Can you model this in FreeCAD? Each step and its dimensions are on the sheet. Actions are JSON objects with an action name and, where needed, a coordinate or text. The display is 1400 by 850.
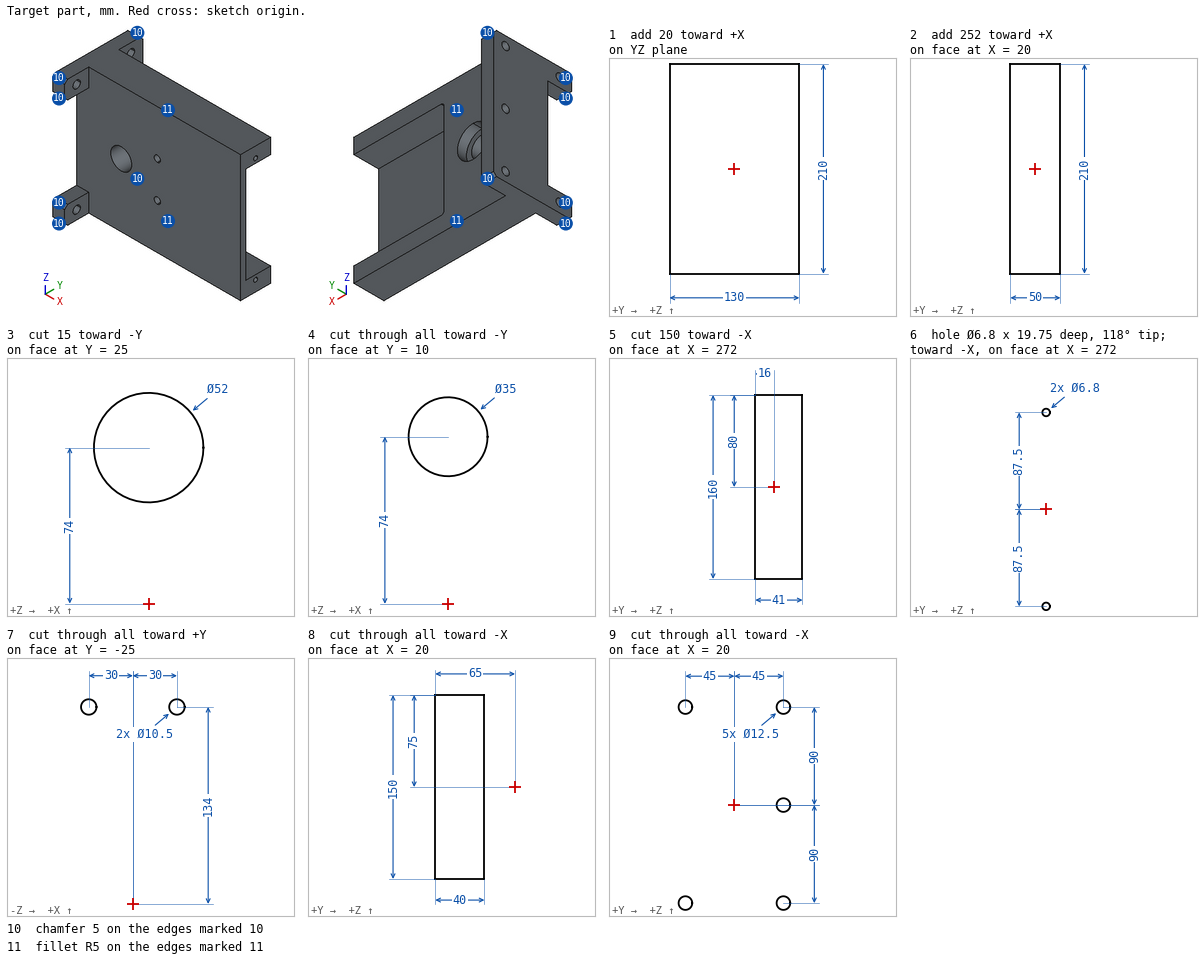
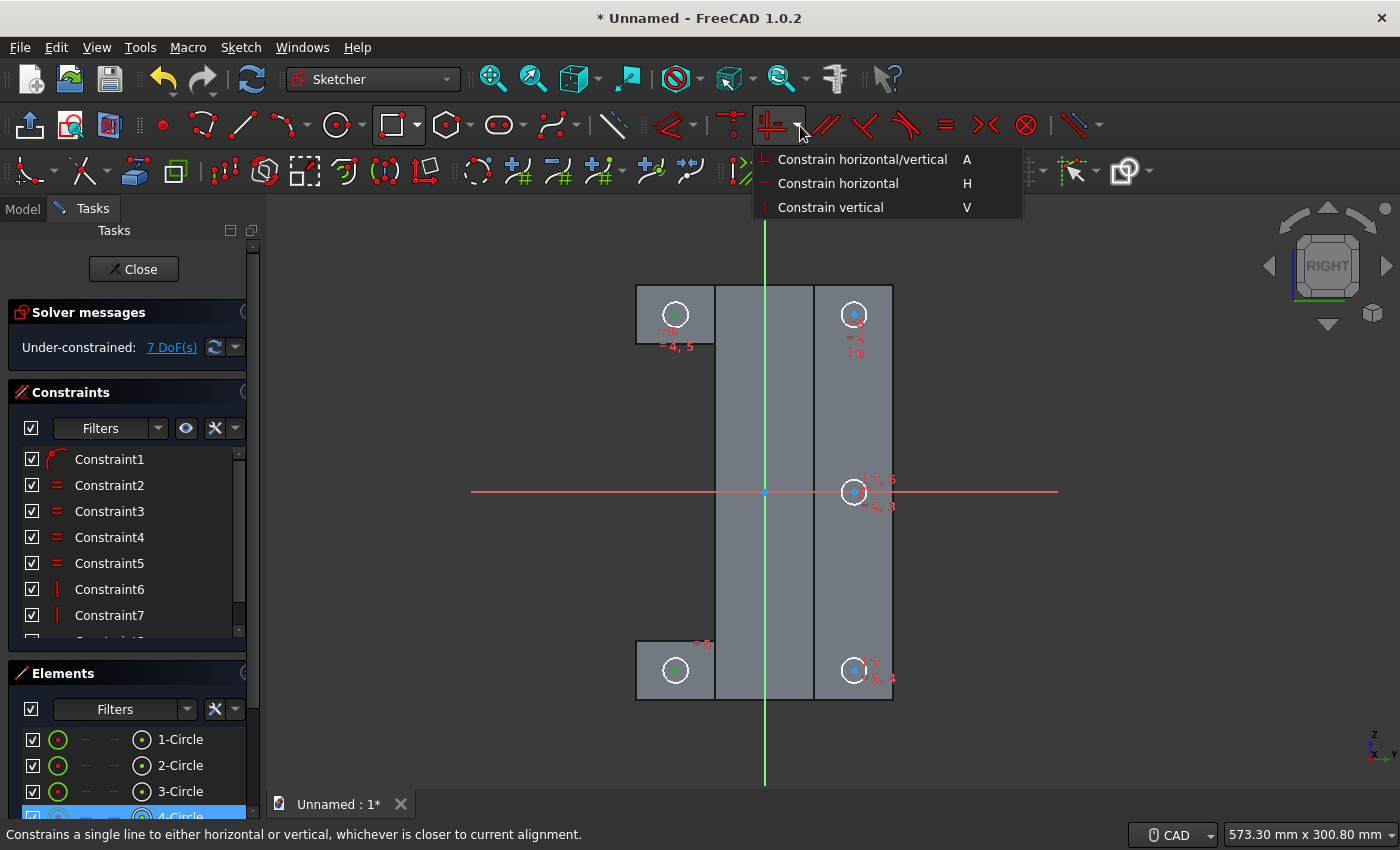
{"action": "left_click", "coordinate": [888, 207]}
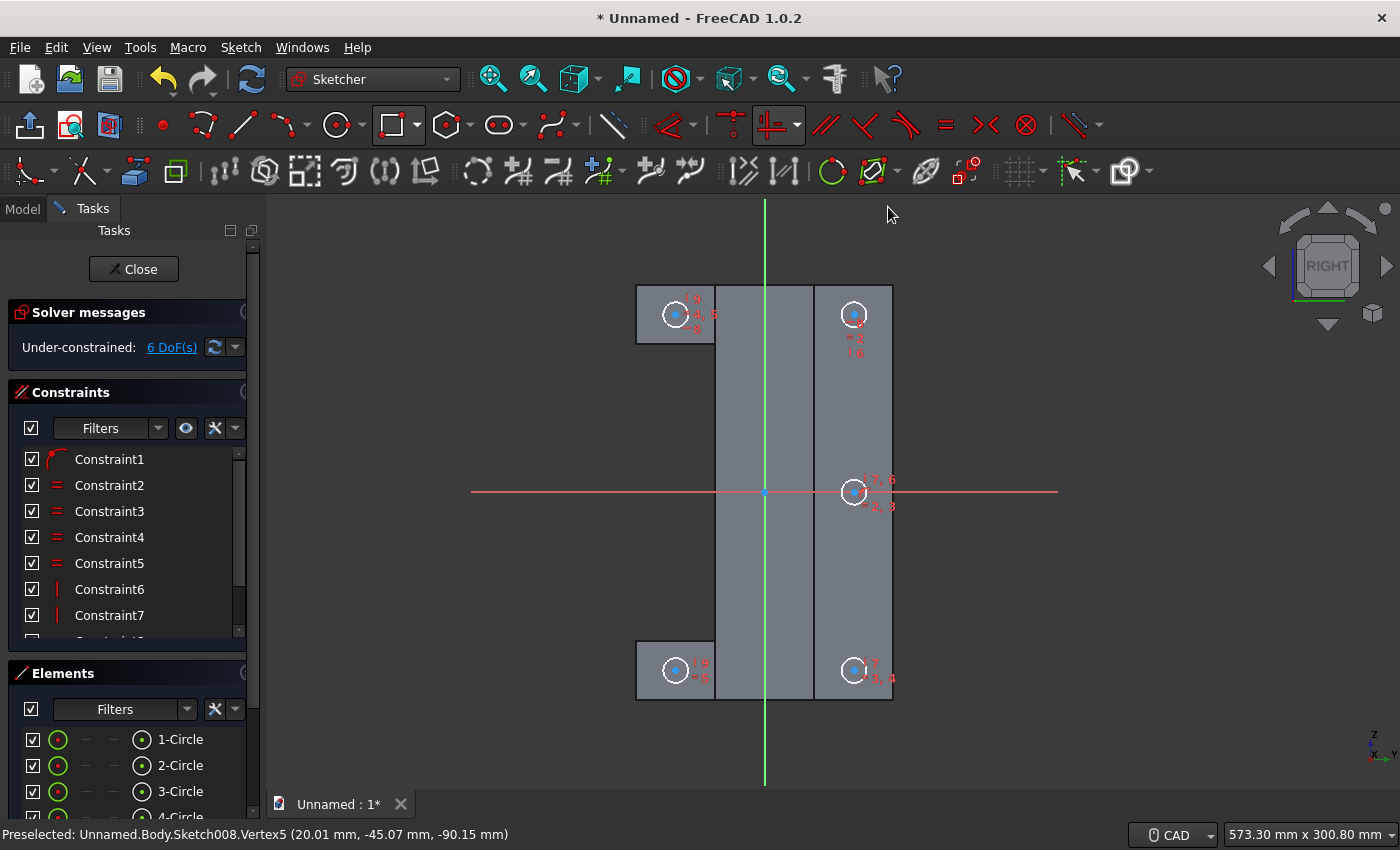
{"action": "left_click", "coordinate": [854, 671]}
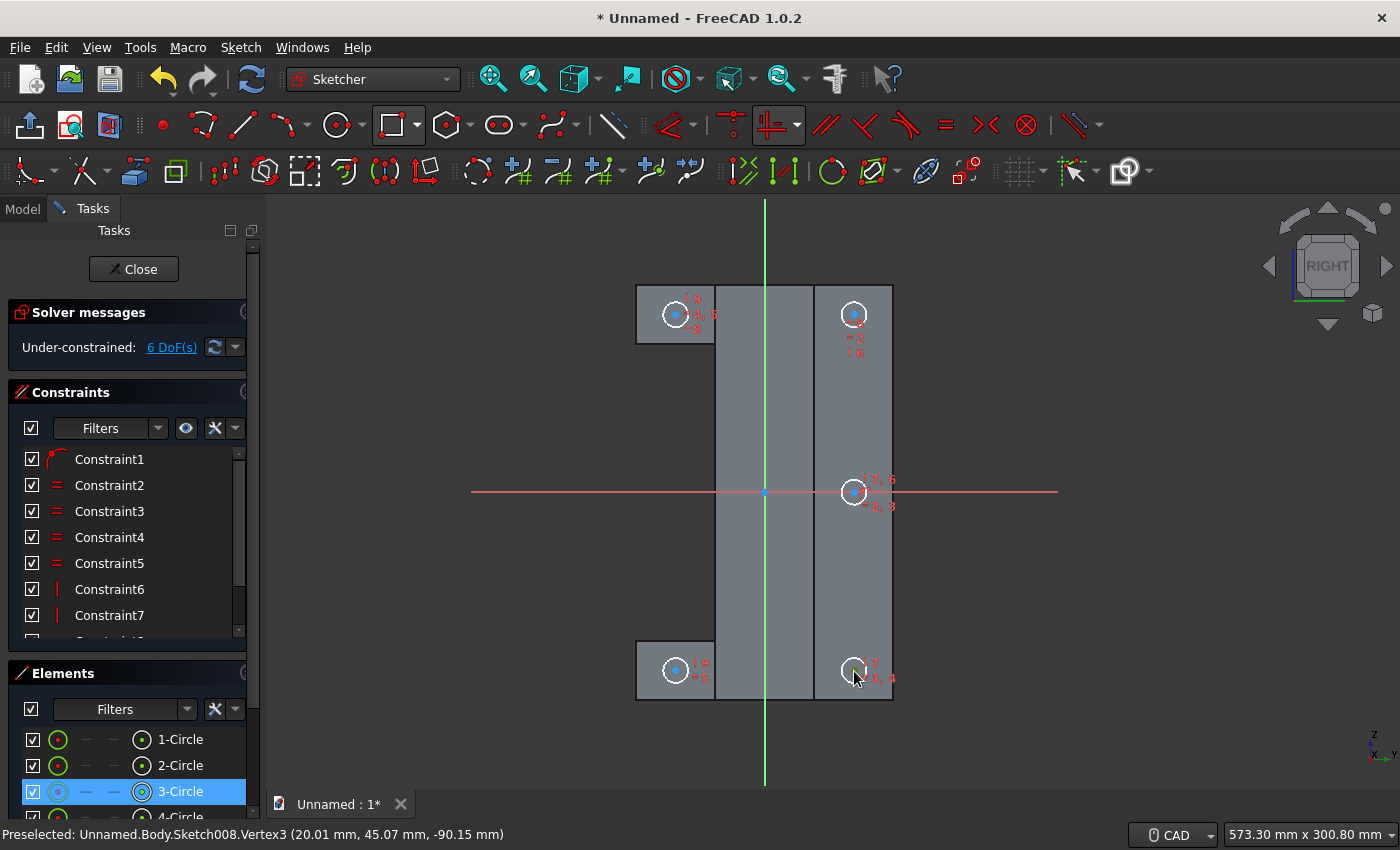
{"action": "left_click", "coordinate": [676, 671]}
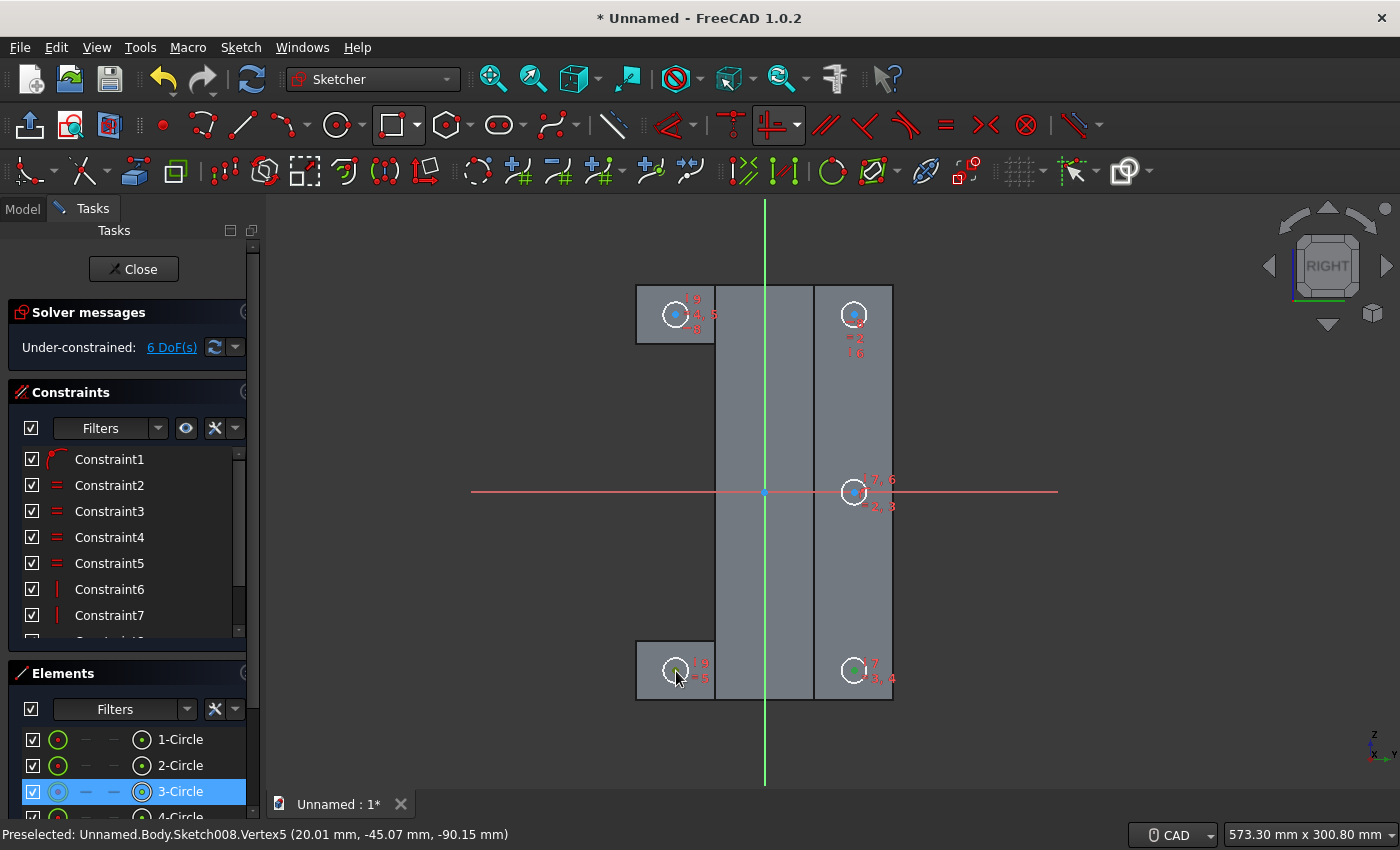
{"action": "left_click", "coordinate": [800, 126]}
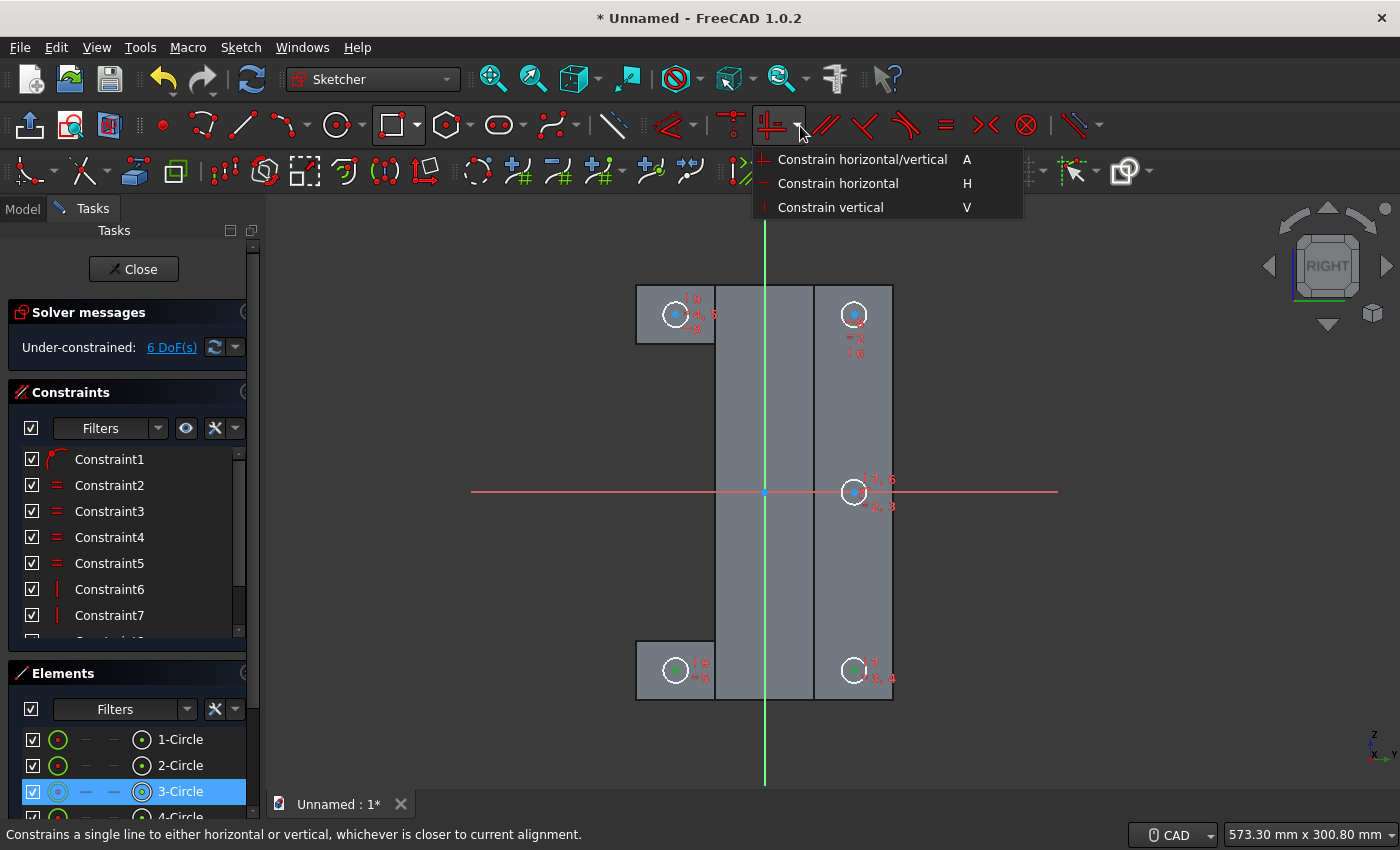
{"action": "left_click", "coordinate": [888, 183]}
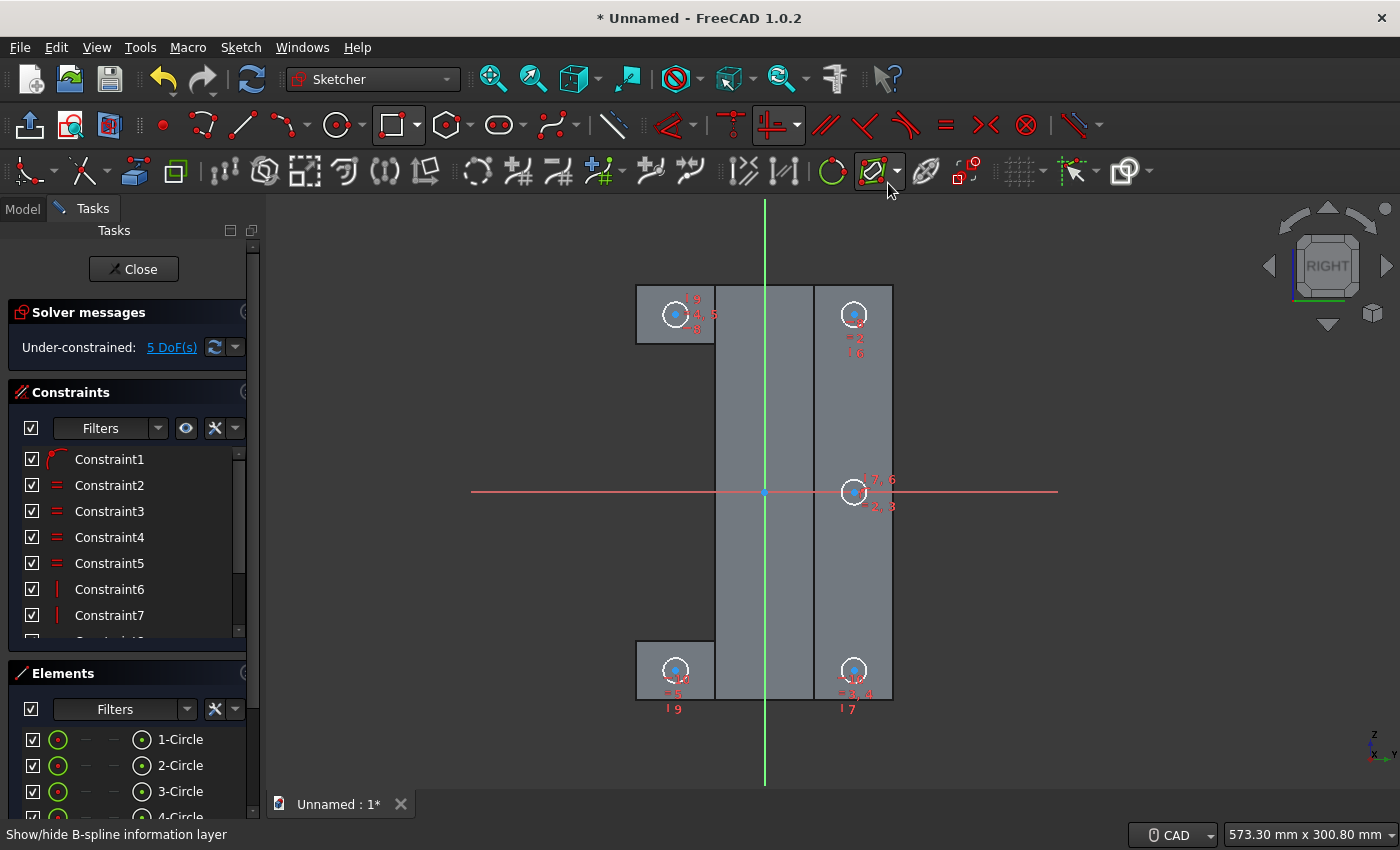
{"action": "left_click", "coordinate": [668, 126]}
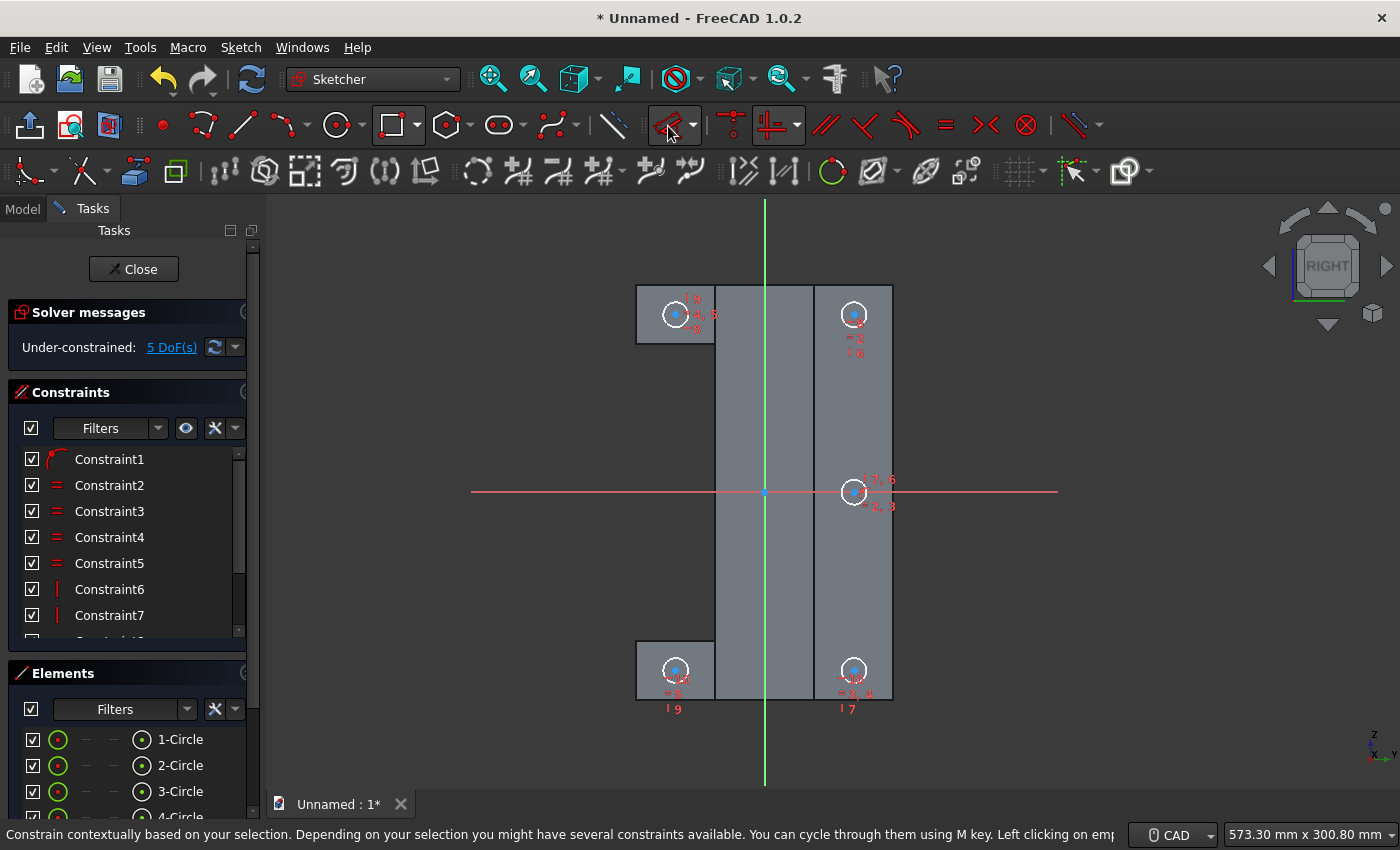
{"action": "scroll", "coordinate": [863, 306], "scroll_direction": "up", "scroll_amount": 3}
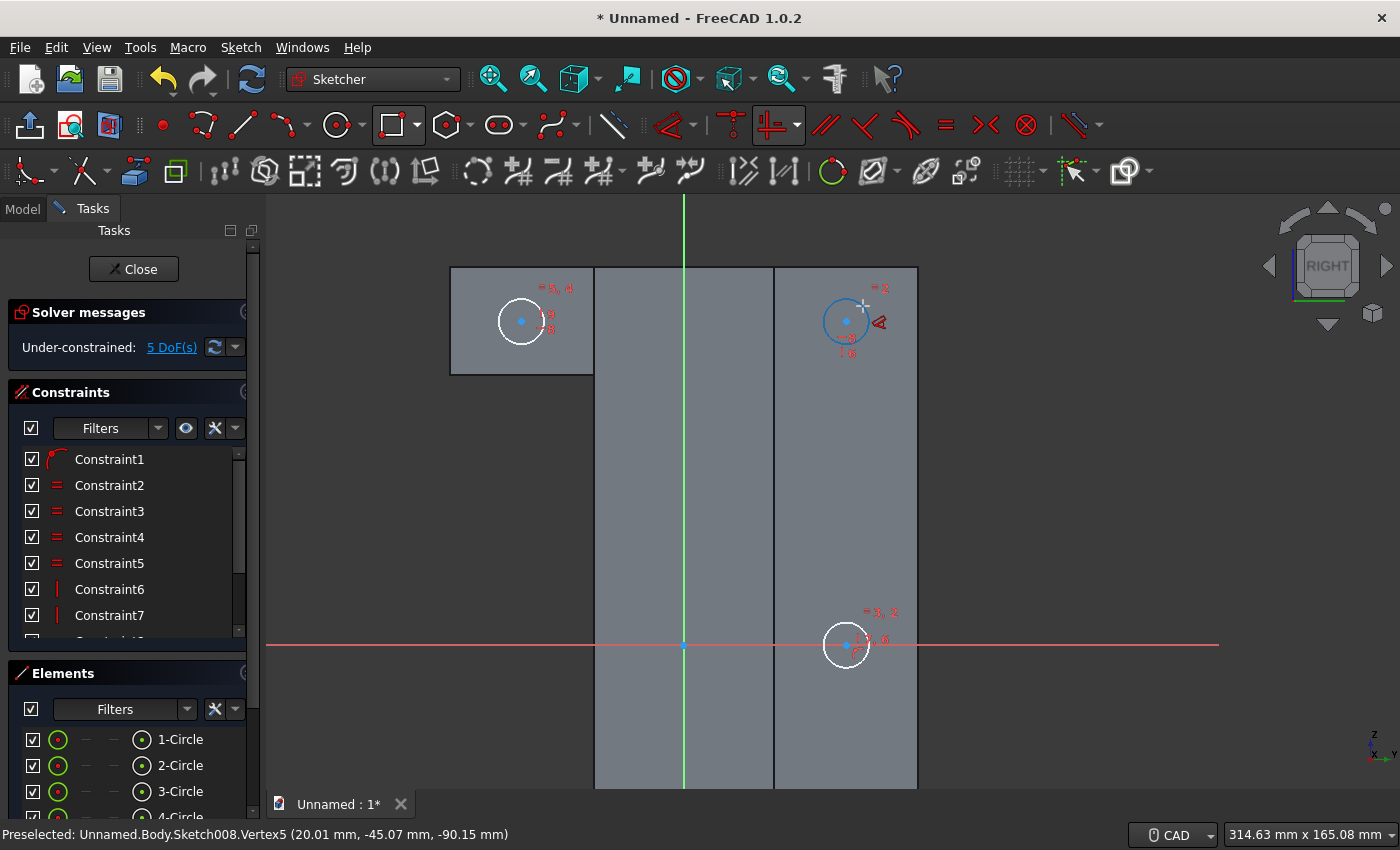
{"action": "left_click", "coordinate": [862, 306]}
{"action": "left_click", "coordinate": [885, 283]}